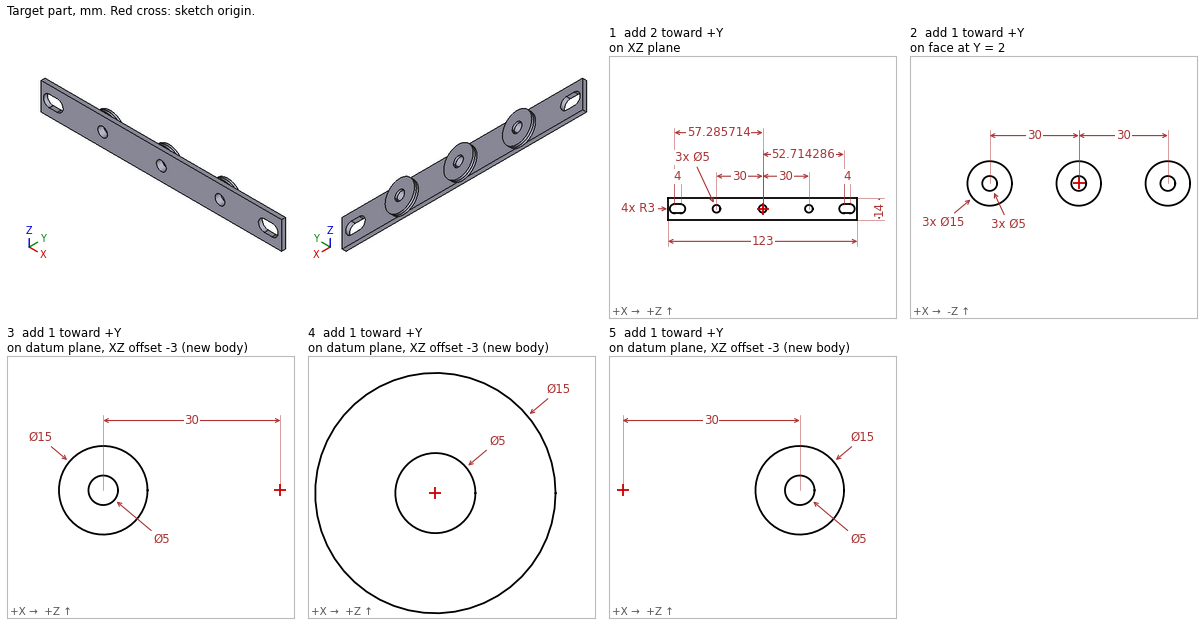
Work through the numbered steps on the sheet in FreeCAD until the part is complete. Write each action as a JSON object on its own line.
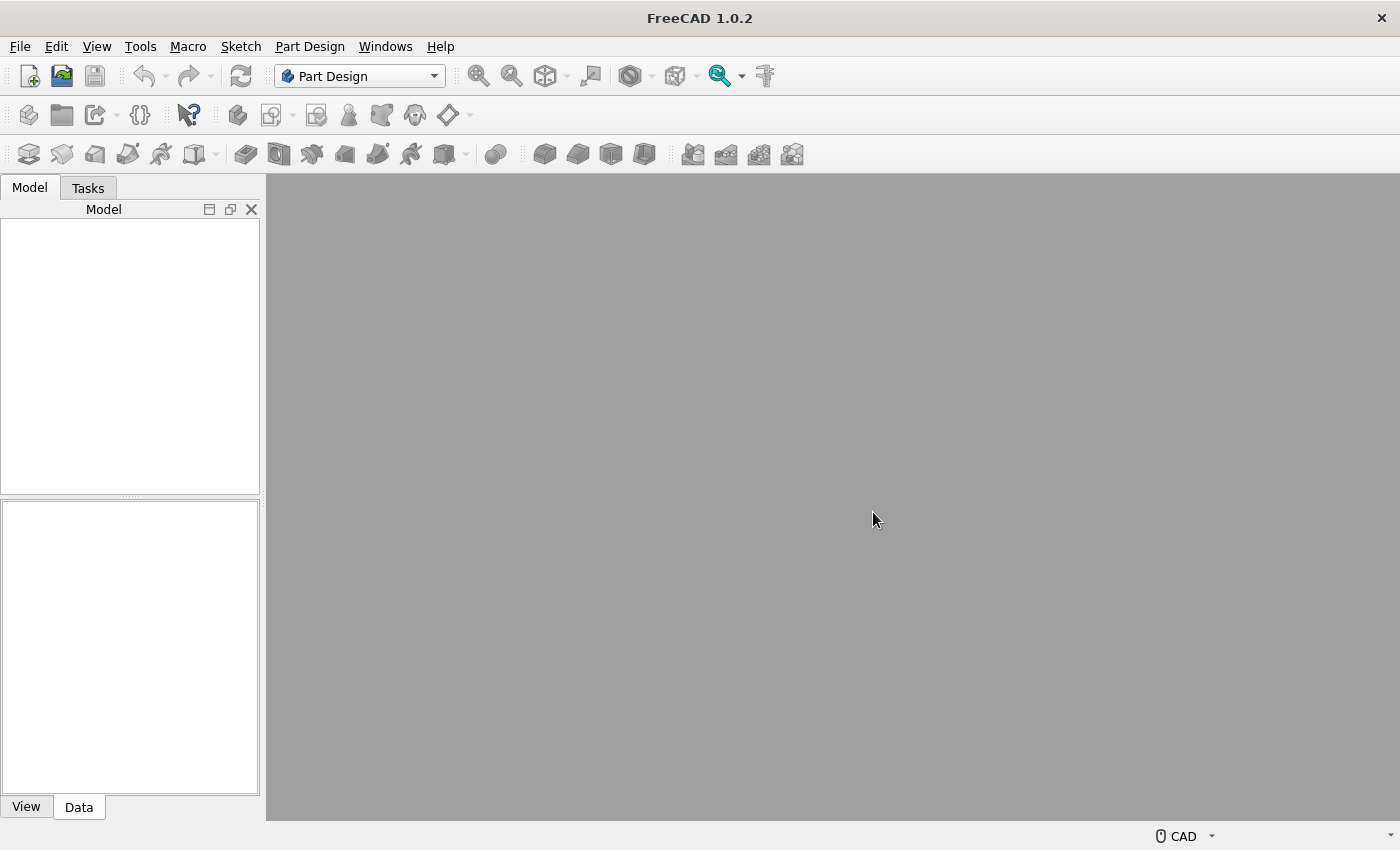
{"action": "left_click", "coordinate": [29, 76]}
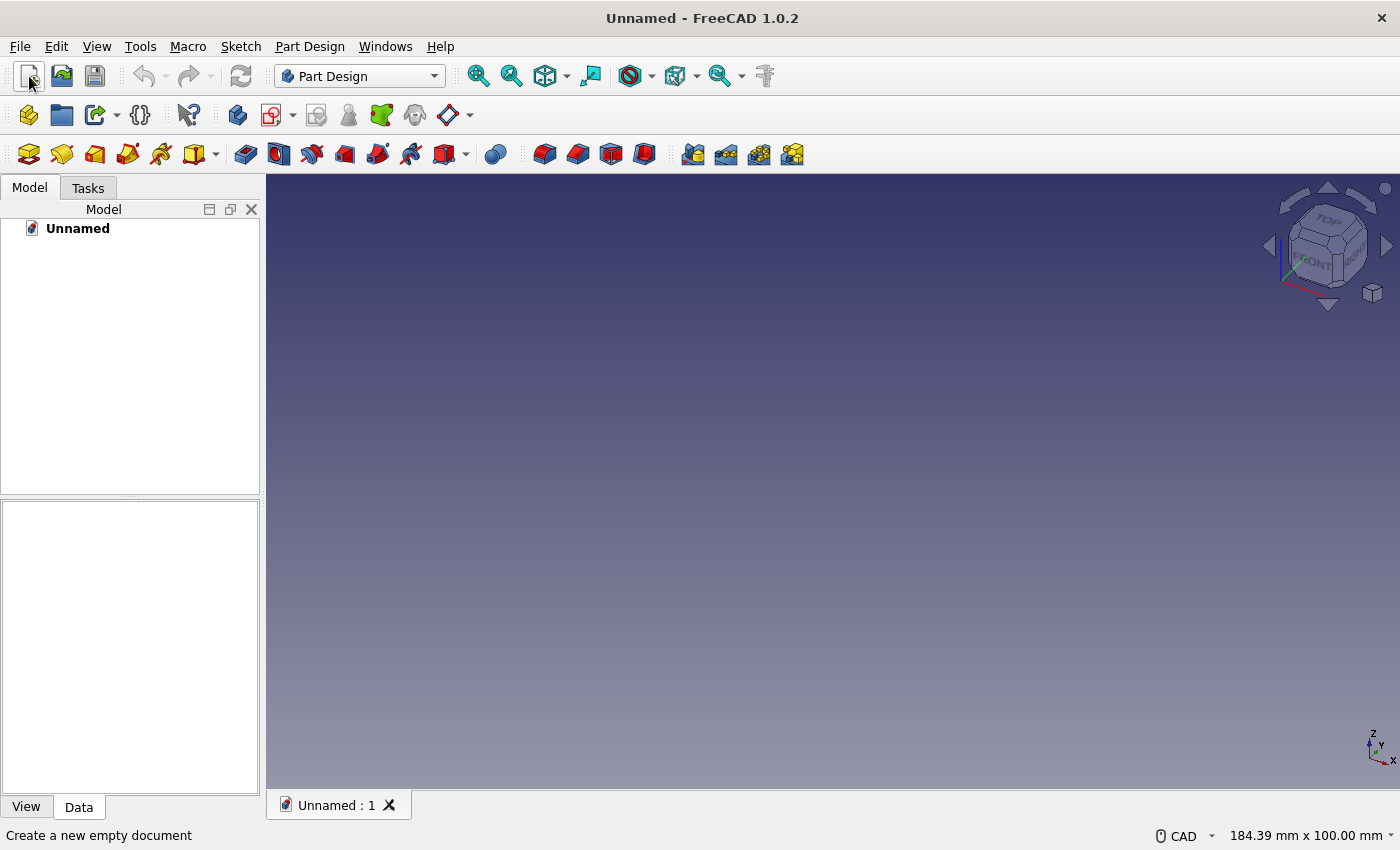
{"action": "left_click", "coordinate": [270, 116]}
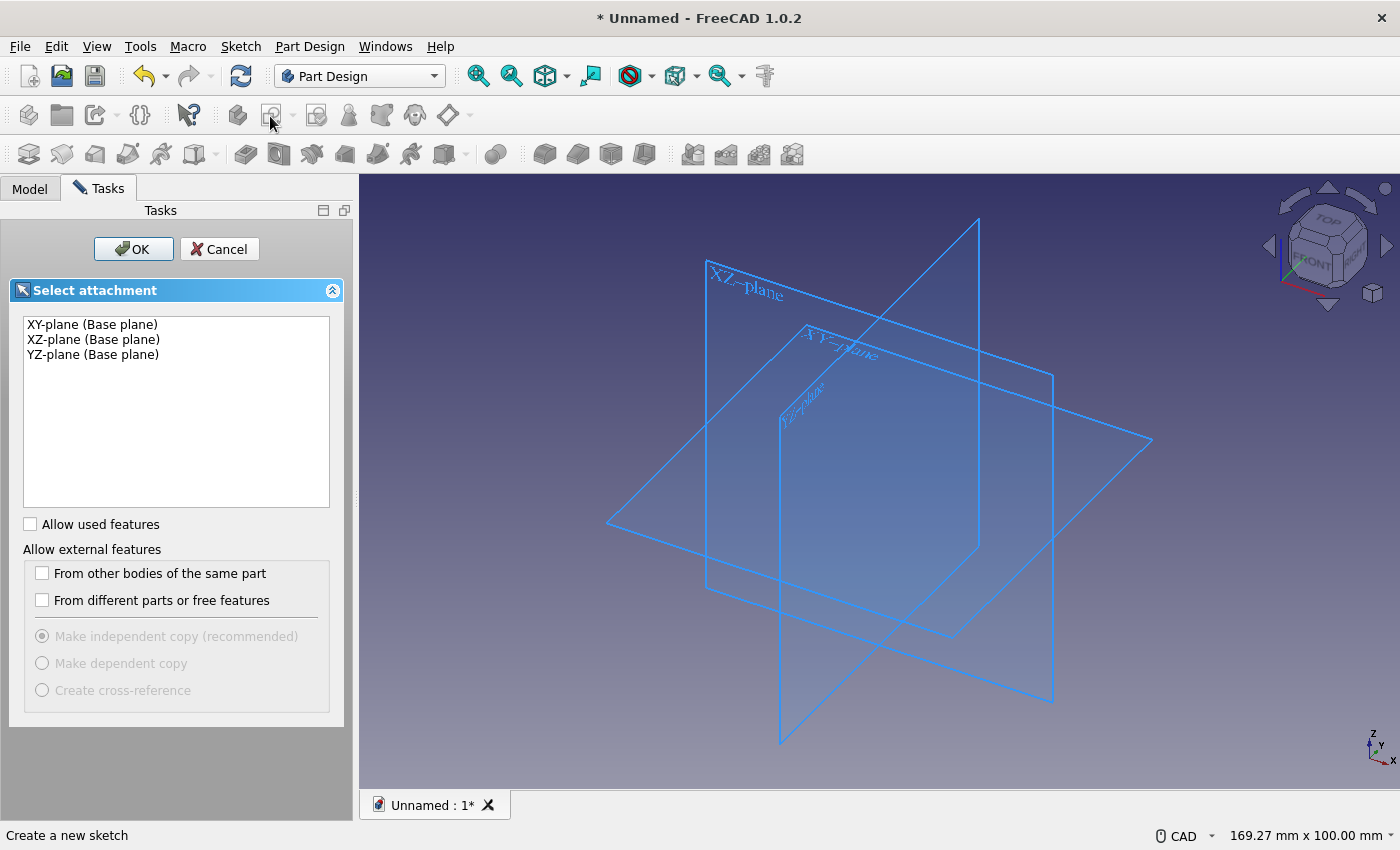
{"action": "left_click", "coordinate": [84, 340]}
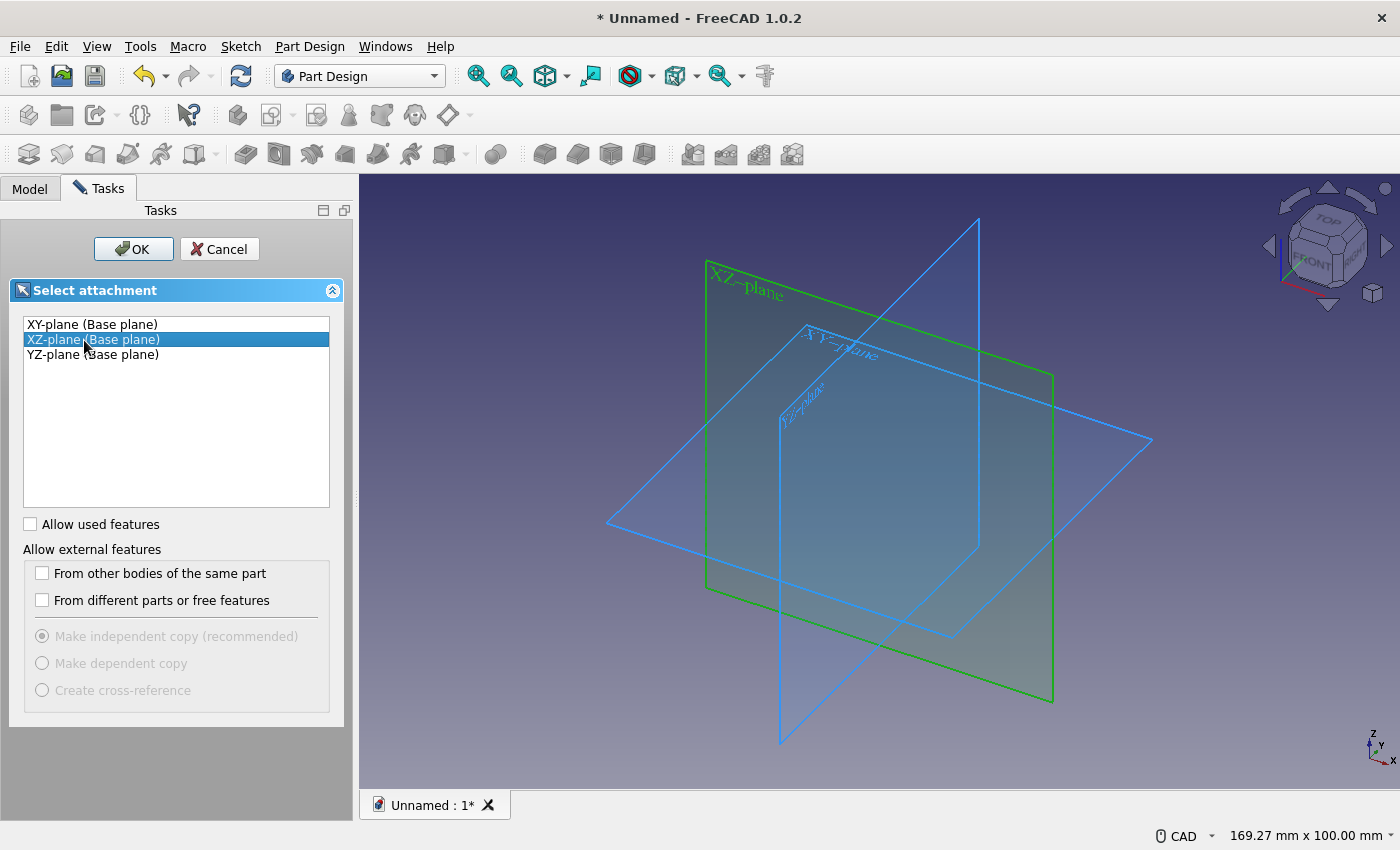
{"action": "left_click", "coordinate": [134, 249]}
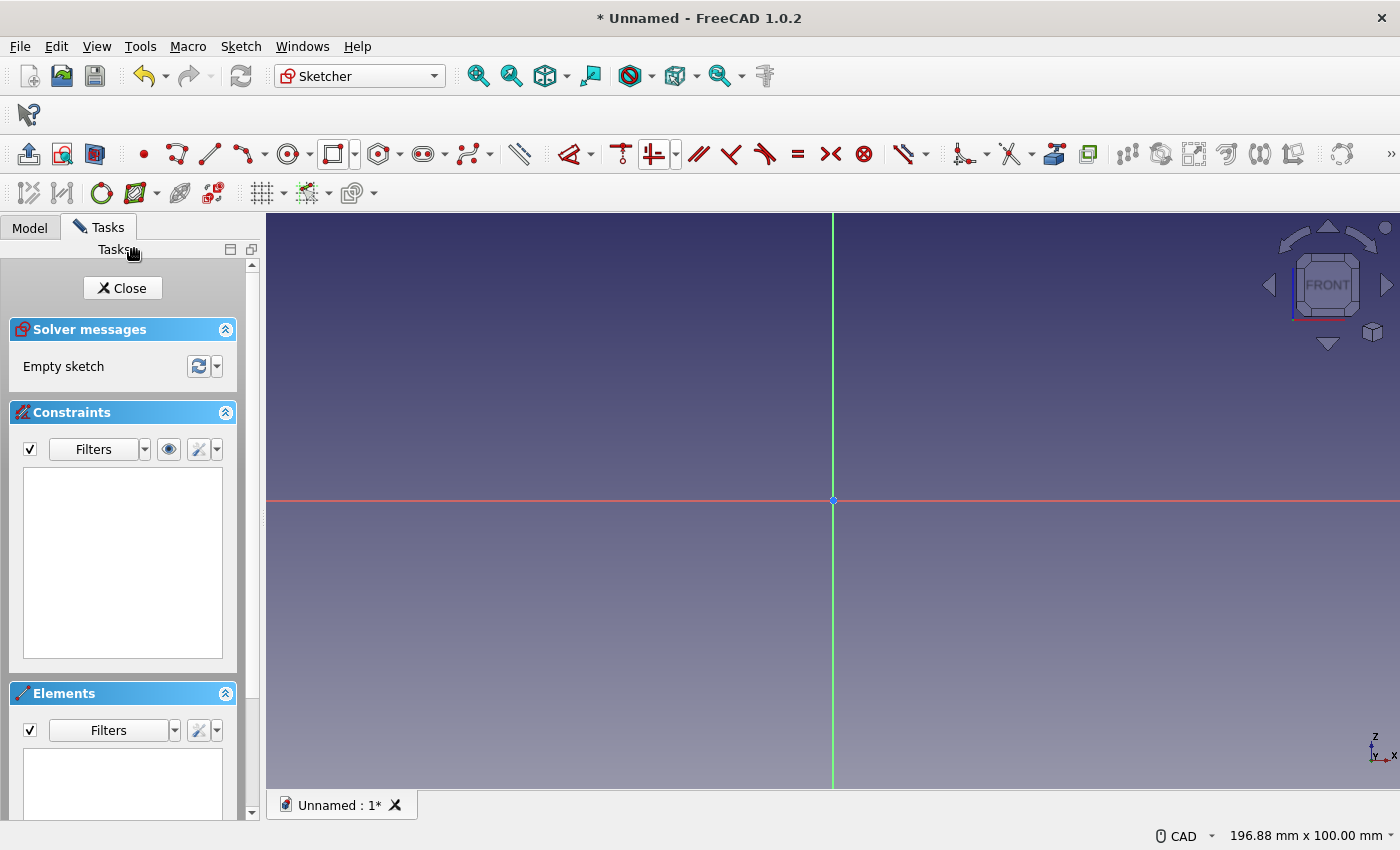
{"action": "left_click", "coordinate": [354, 154]}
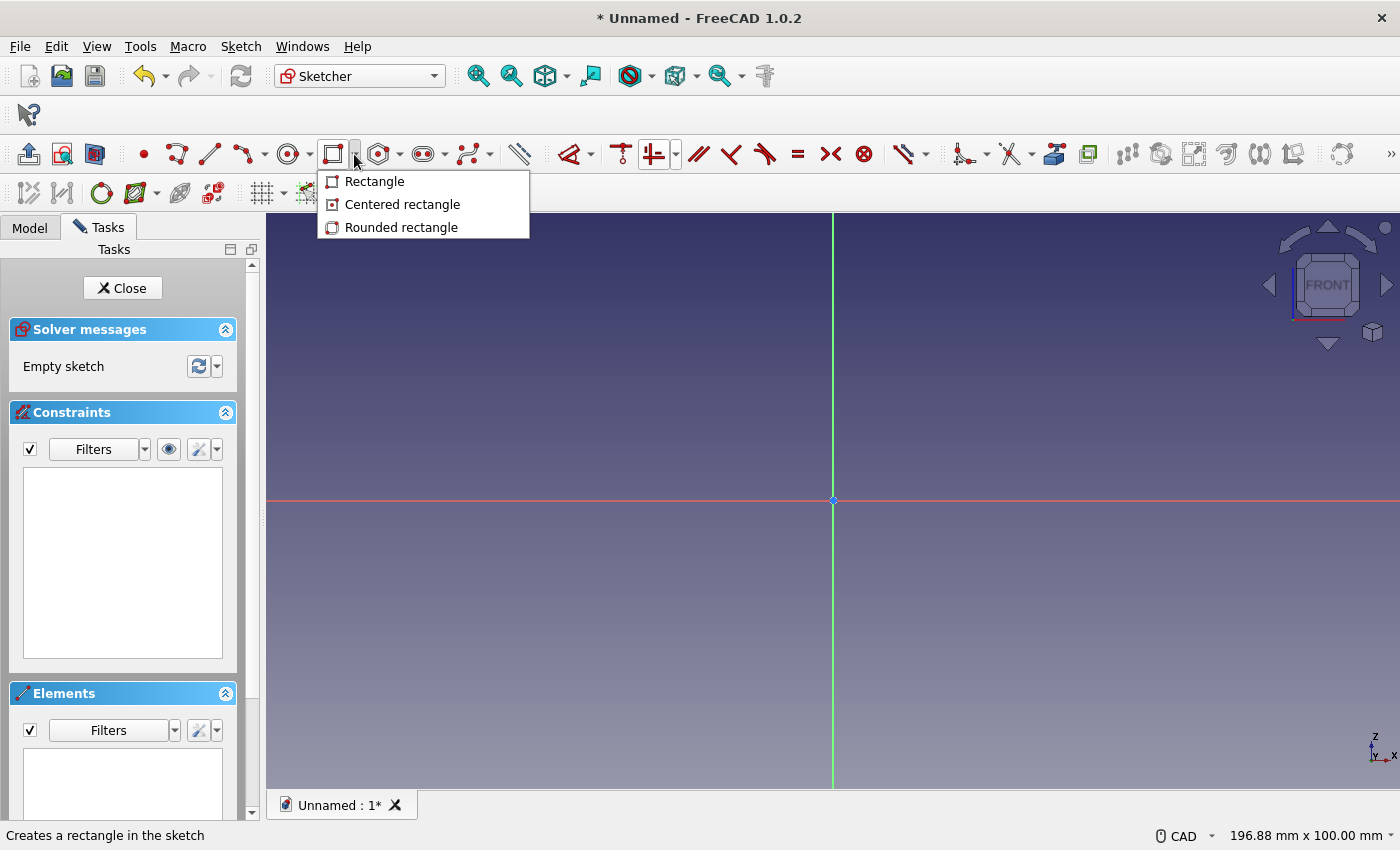
{"action": "left_click", "coordinate": [424, 204]}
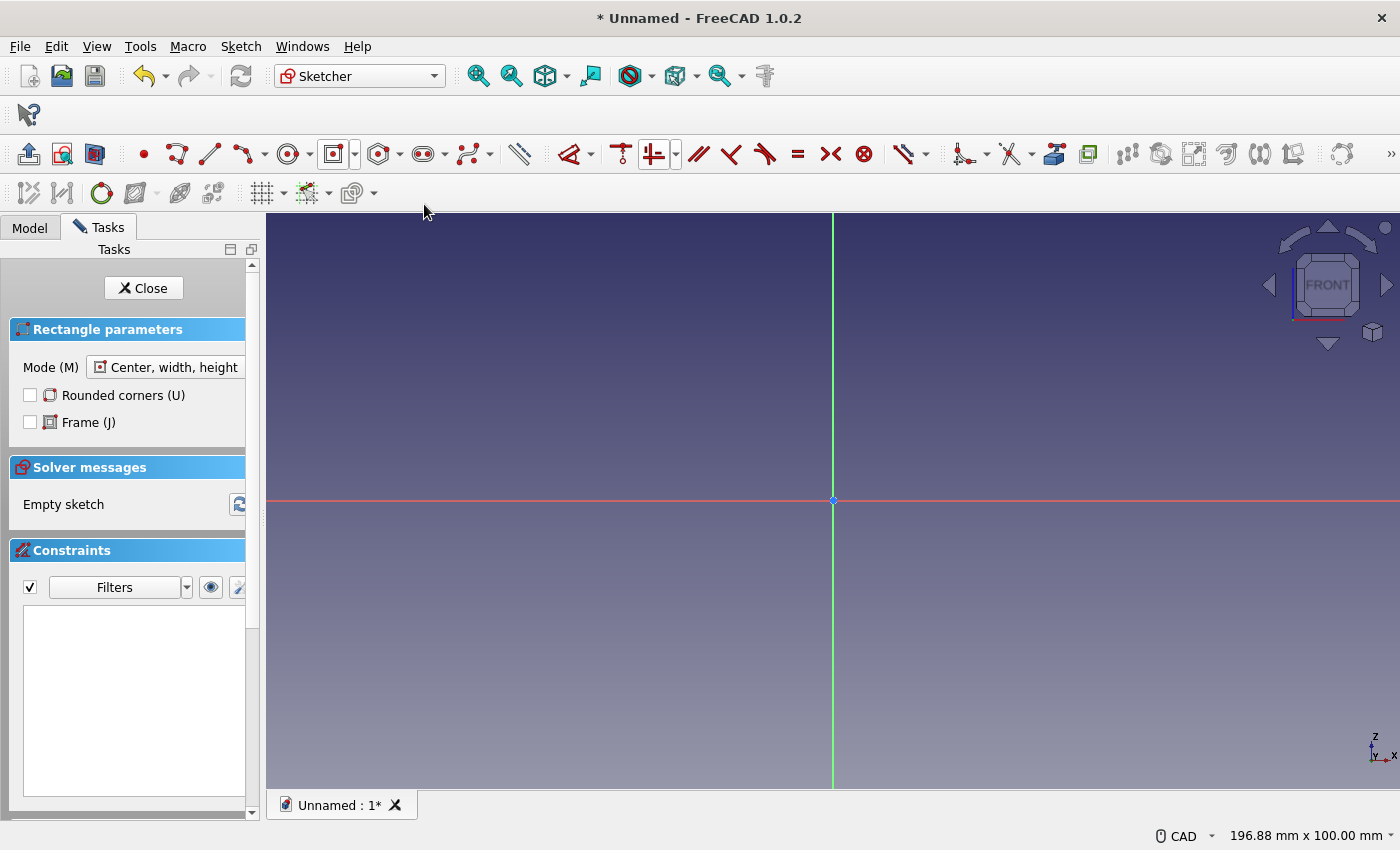
{"action": "left_click", "coordinate": [833, 501]}
{"action": "left_click", "coordinate": [1187, 461]}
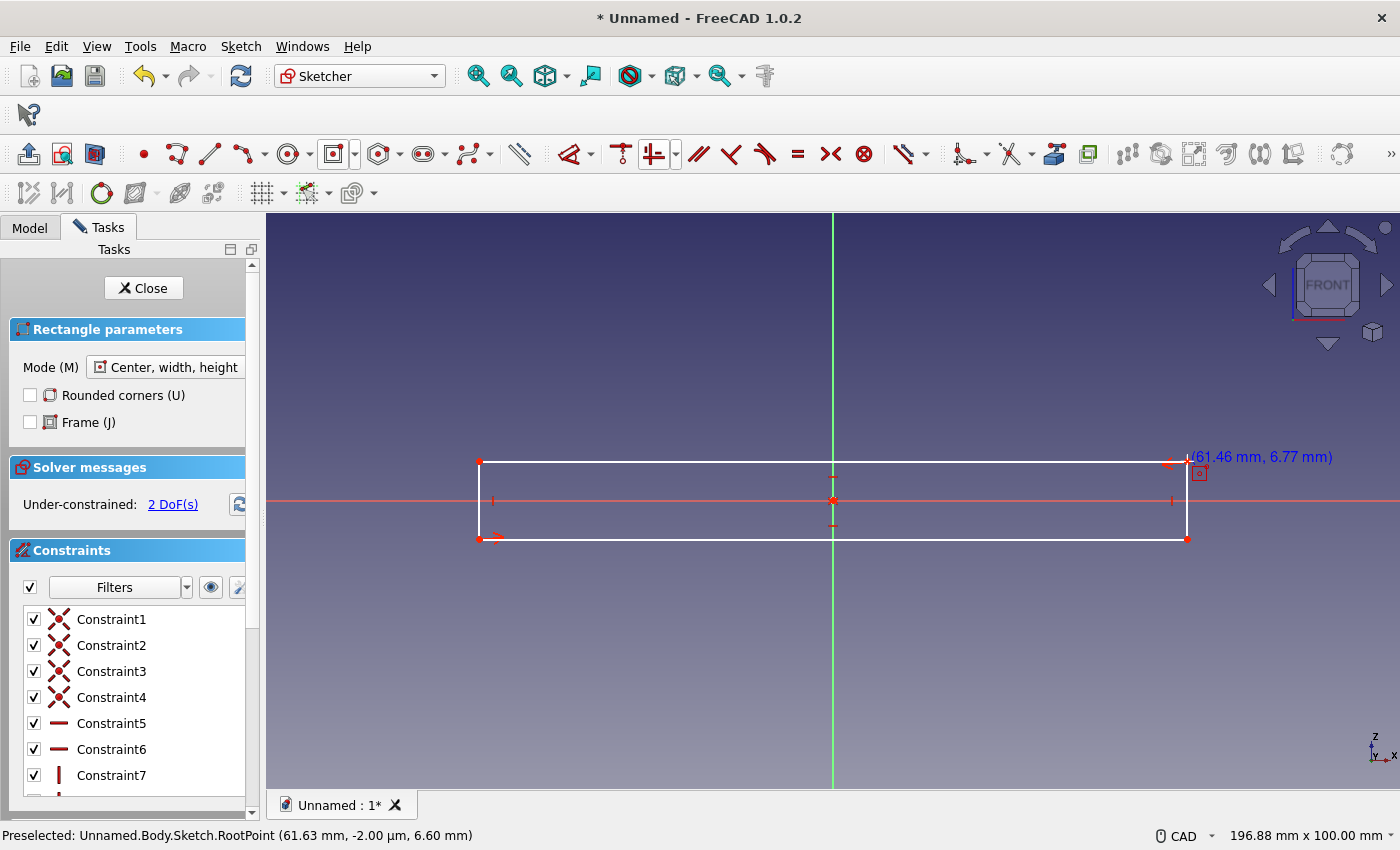
{"action": "left_click", "coordinate": [422, 154]}